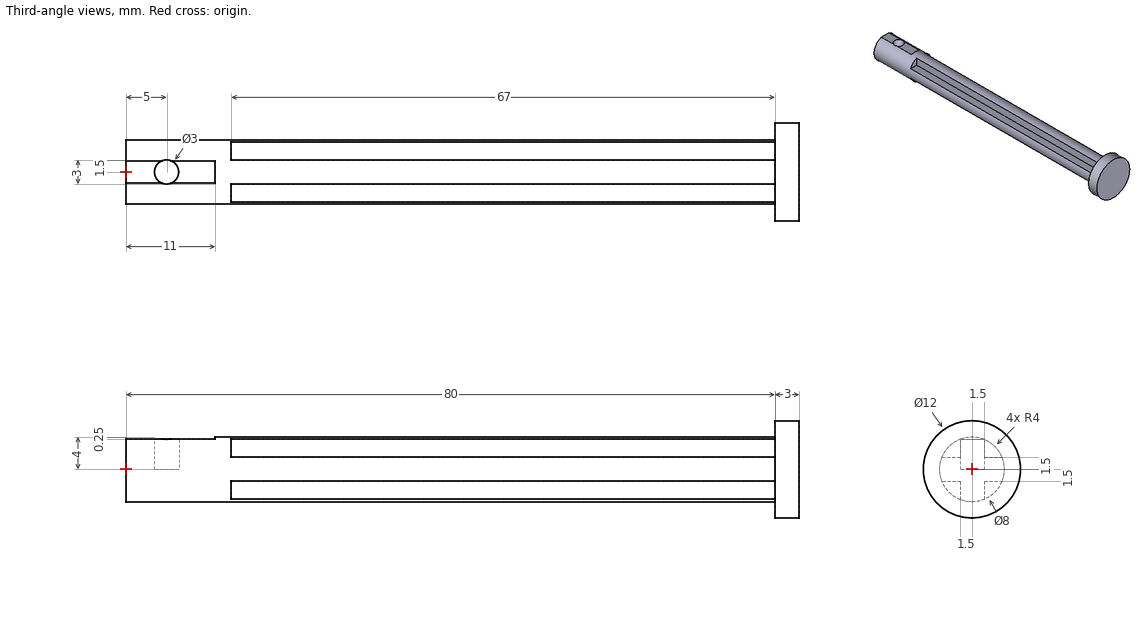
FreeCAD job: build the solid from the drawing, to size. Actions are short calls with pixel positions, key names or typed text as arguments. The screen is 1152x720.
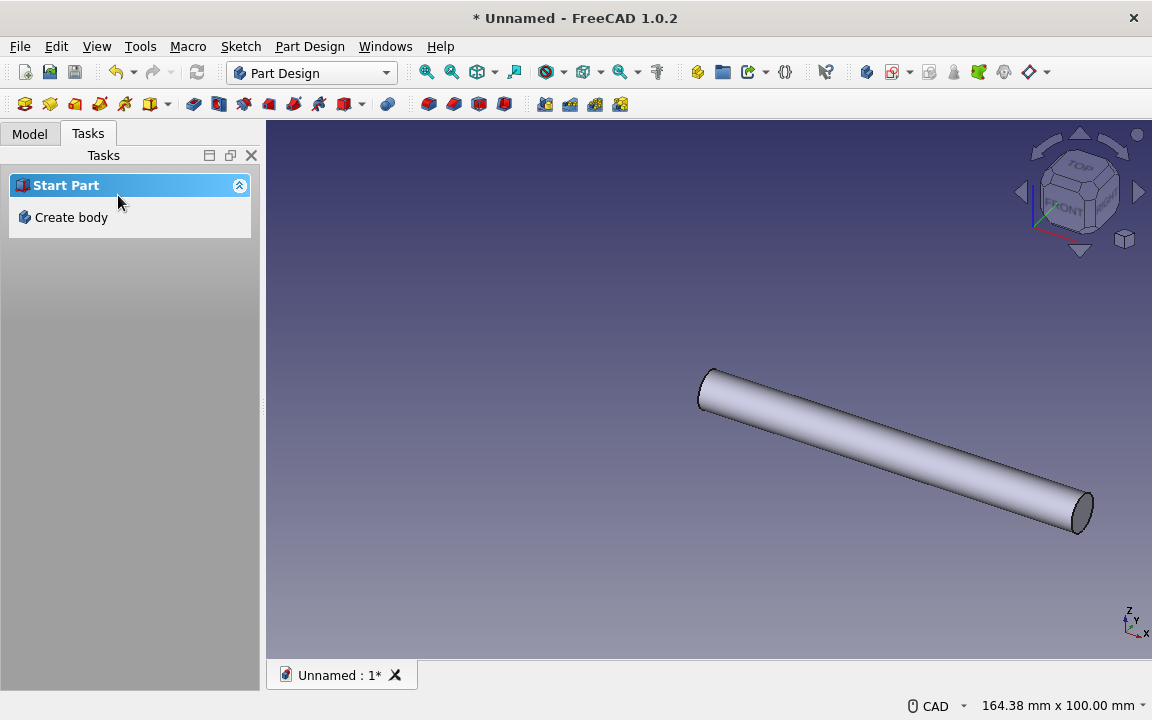
click(427, 72)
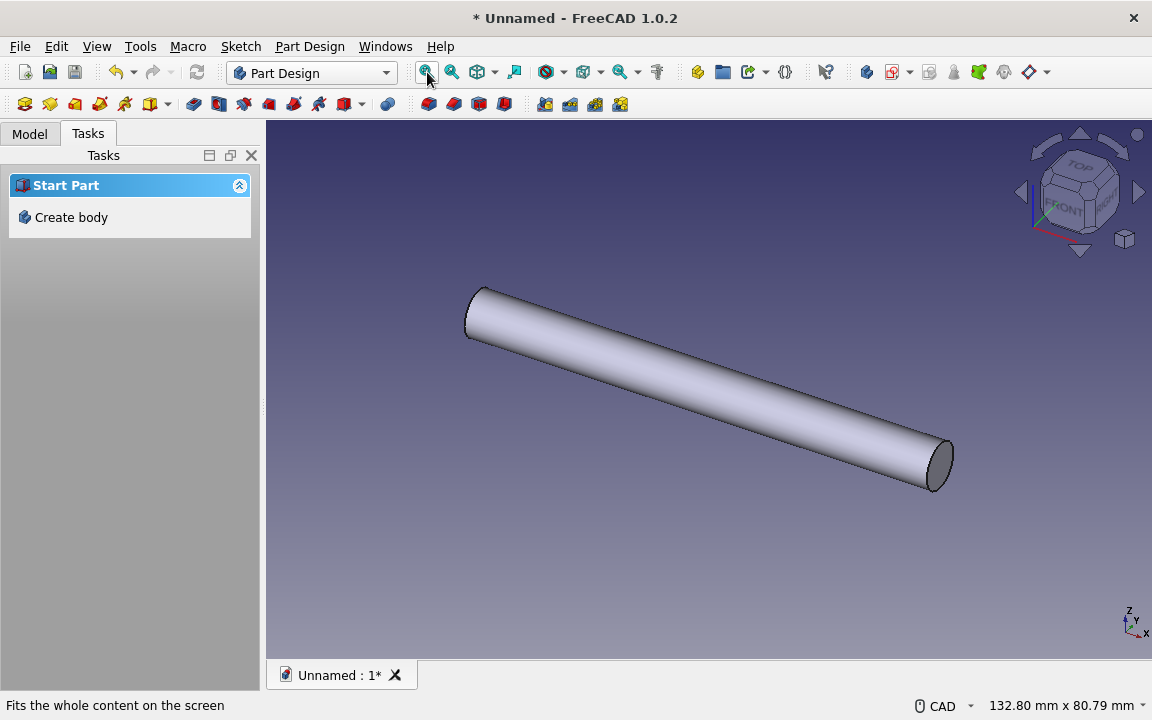
click(30, 134)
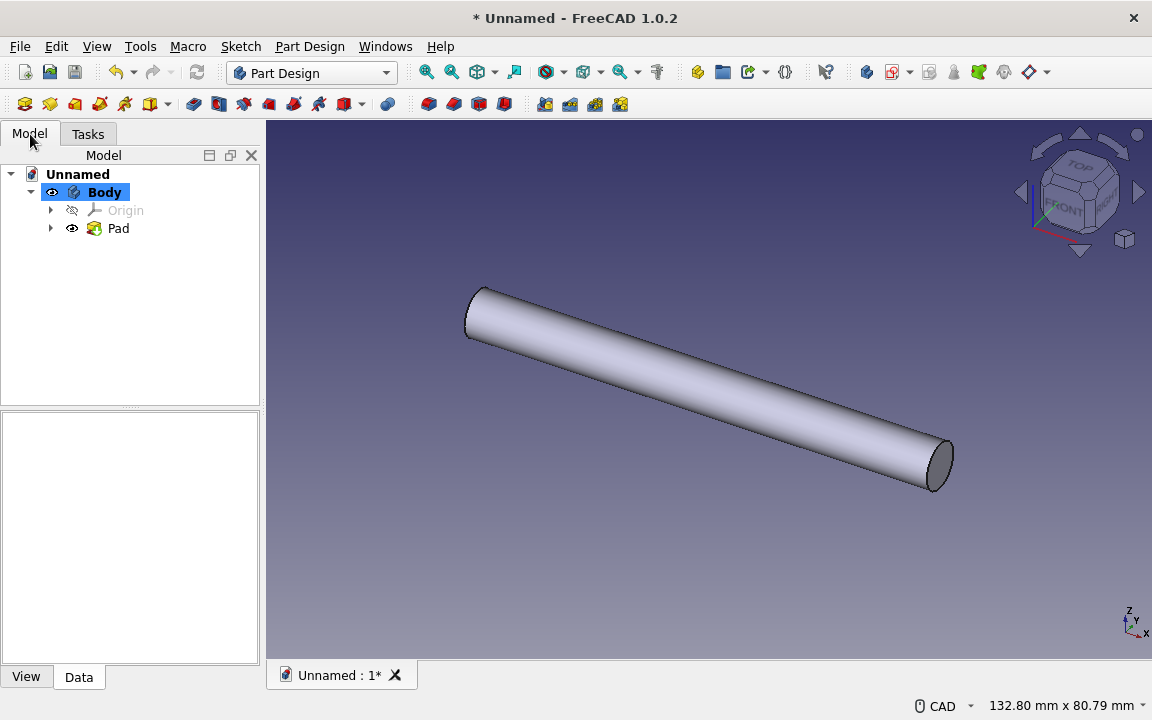
click(51, 210)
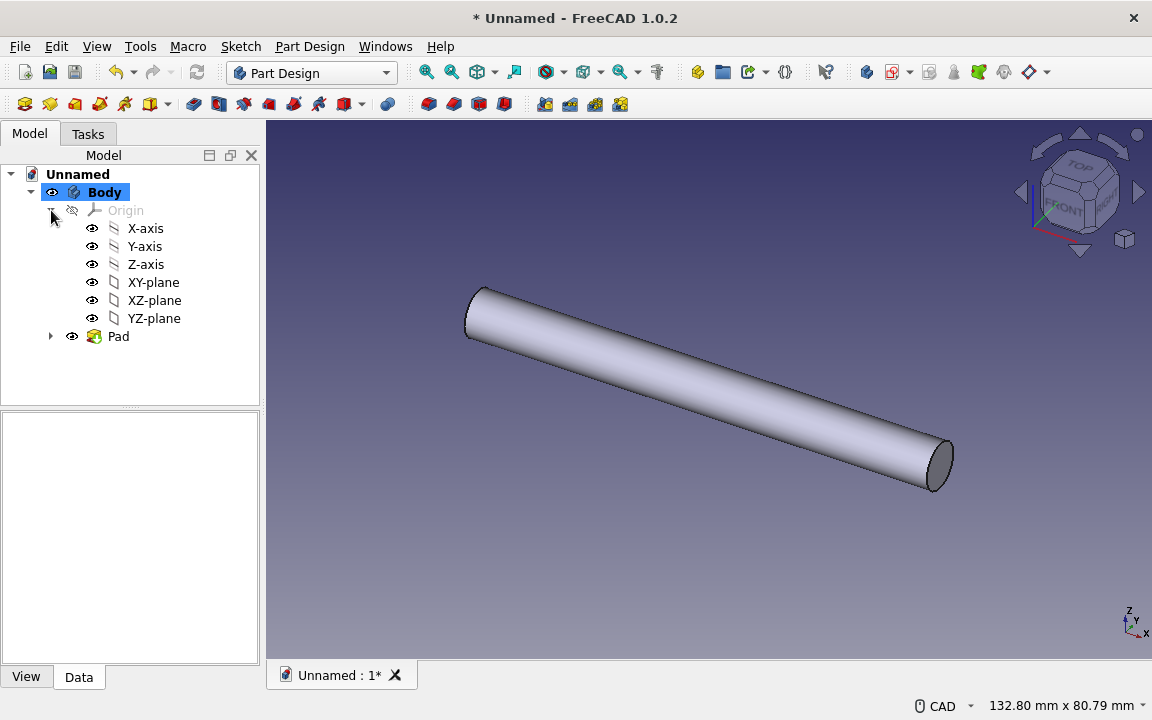
click(137, 318)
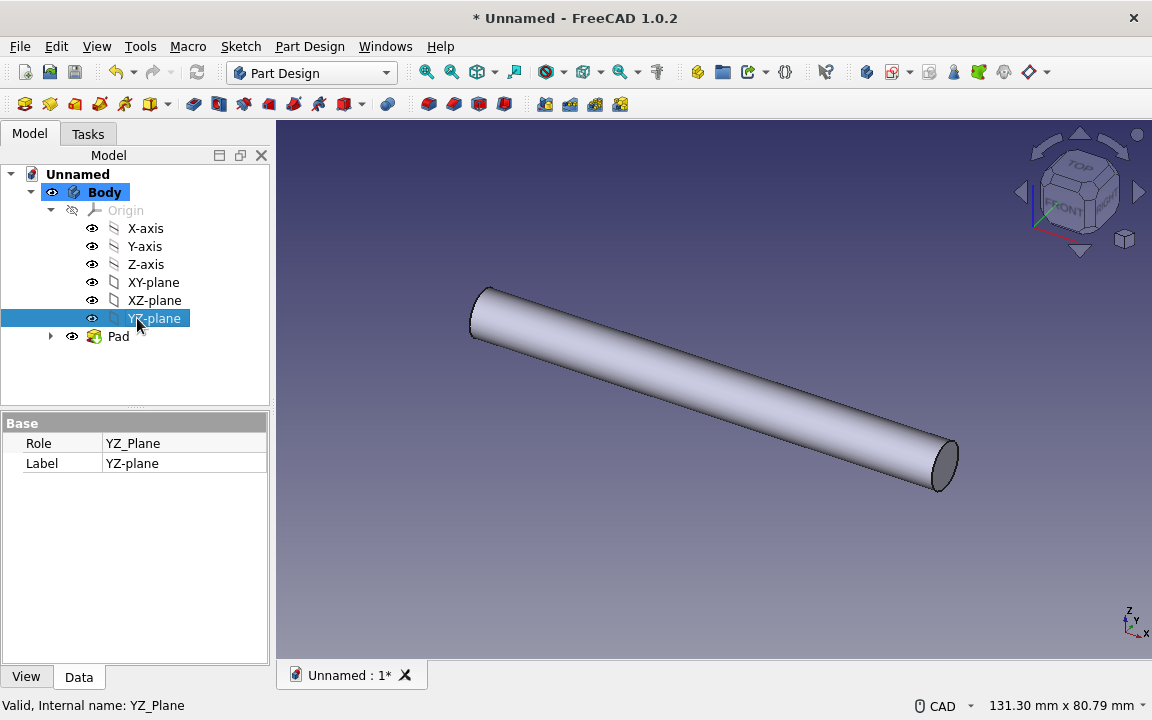
click(1028, 72)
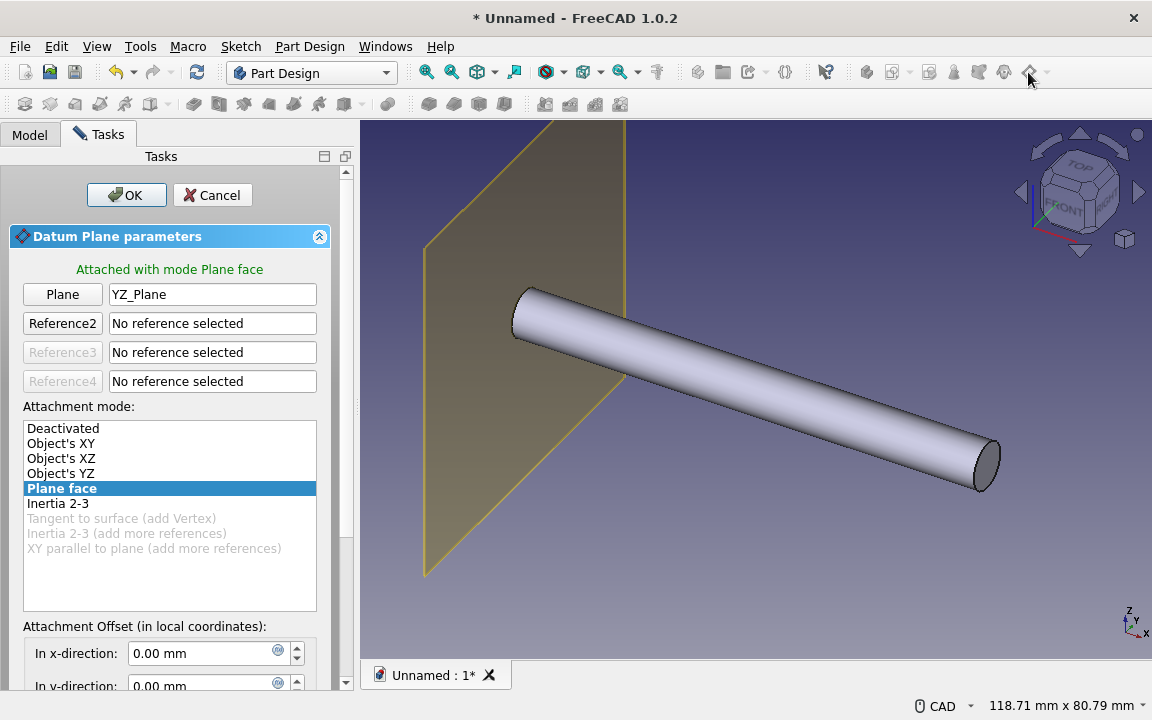
scroll(346, 428, down, 2)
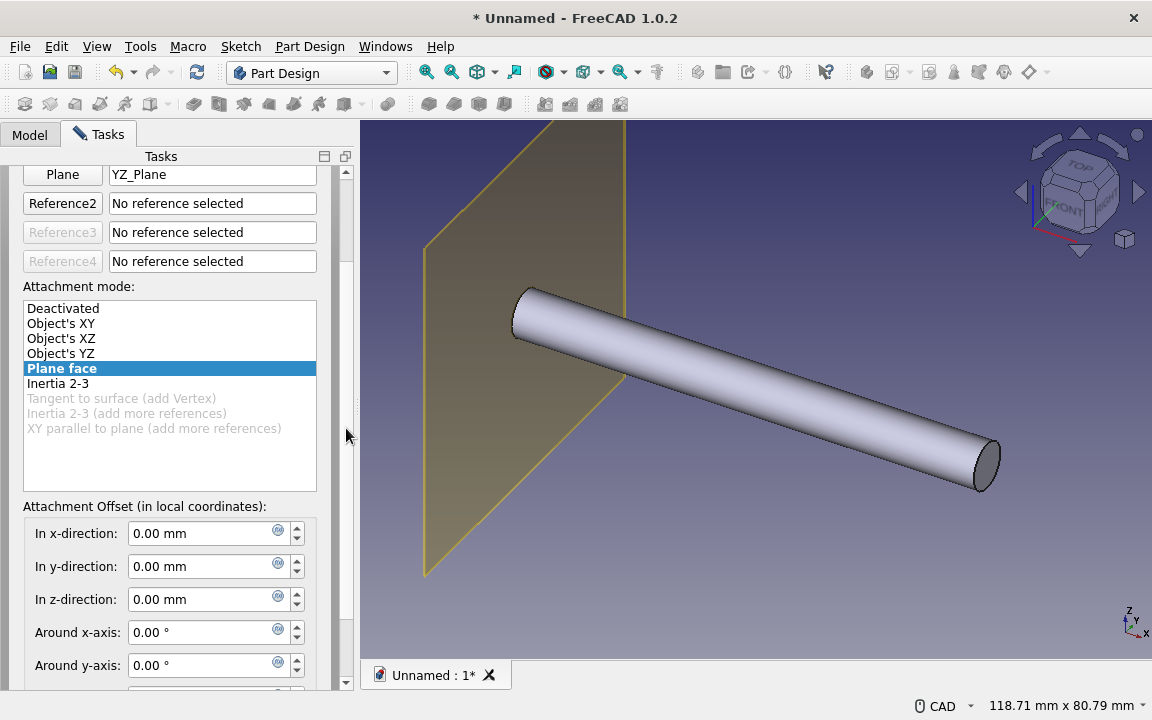
triple_click(210, 600)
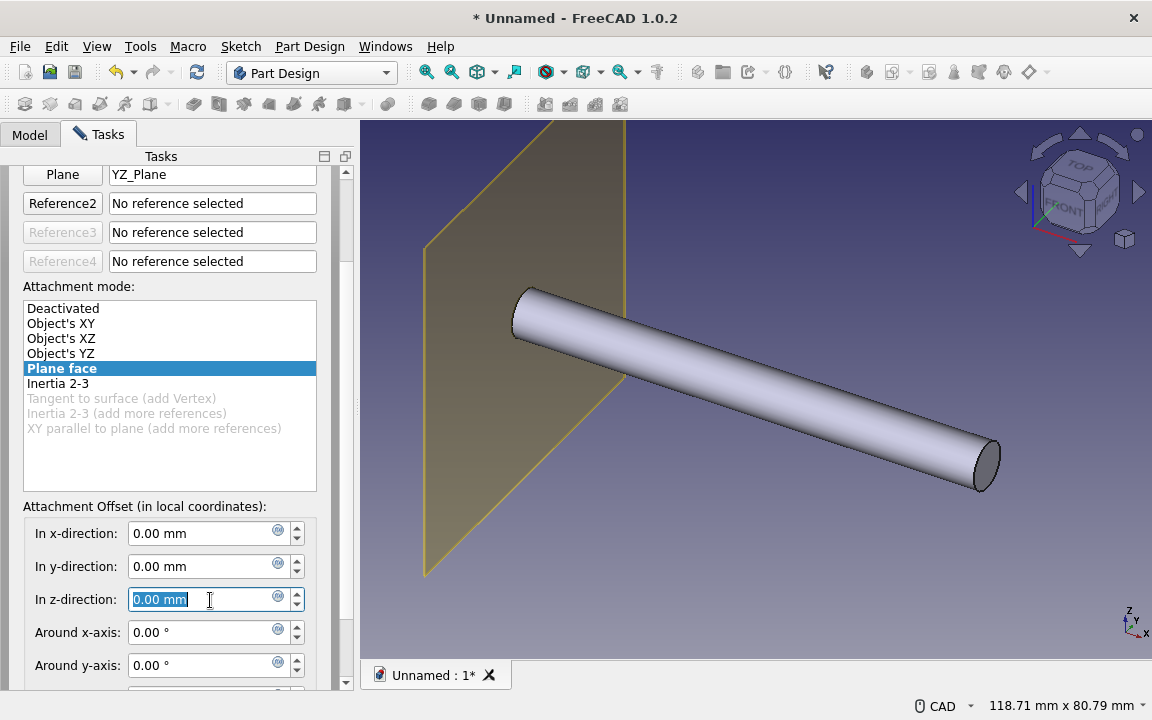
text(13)
key(Tab)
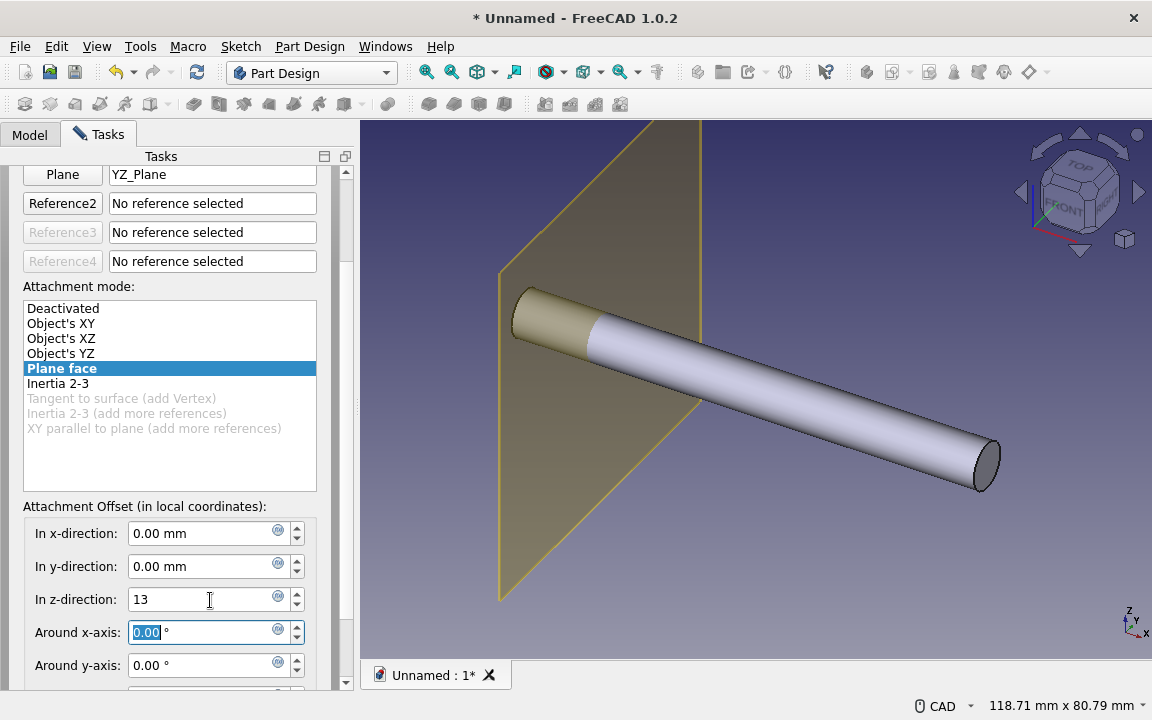
scroll(346, 428, up, 3)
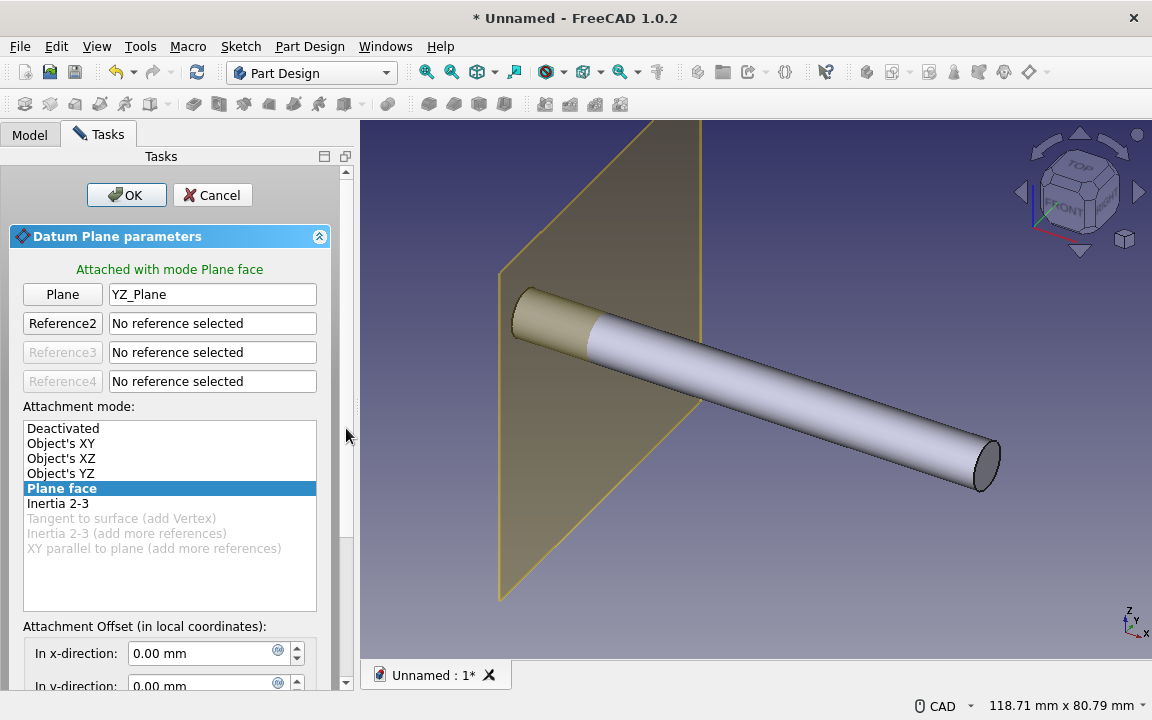
click(127, 195)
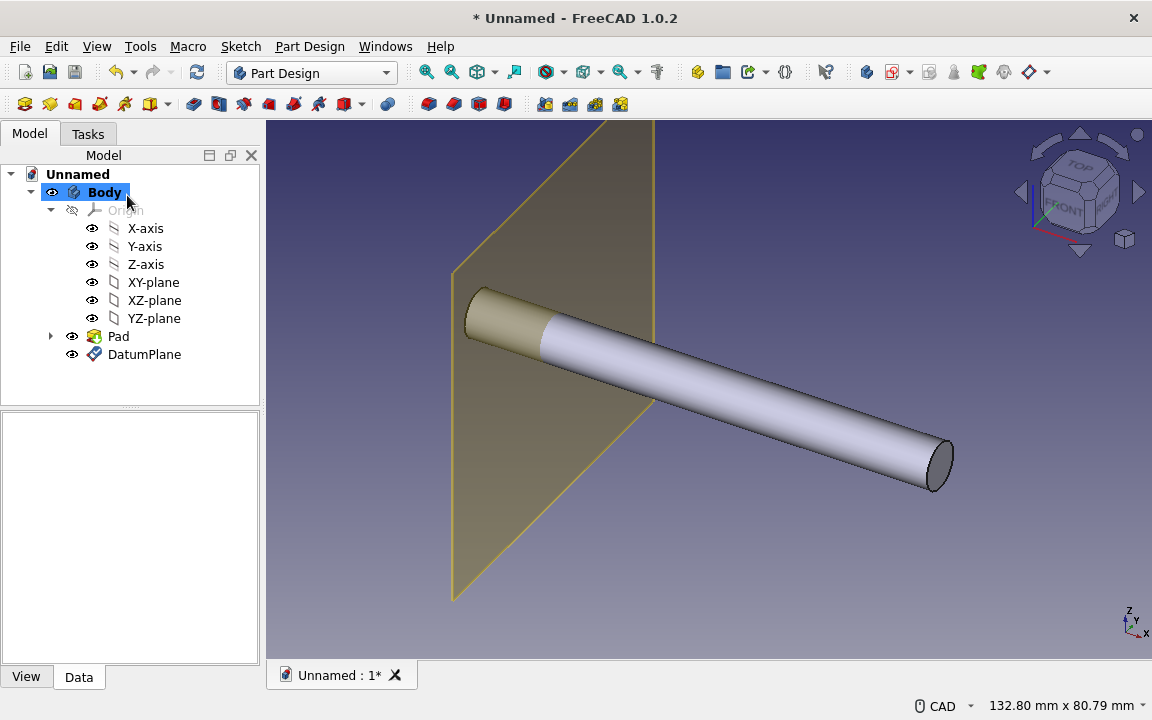
click(117, 354)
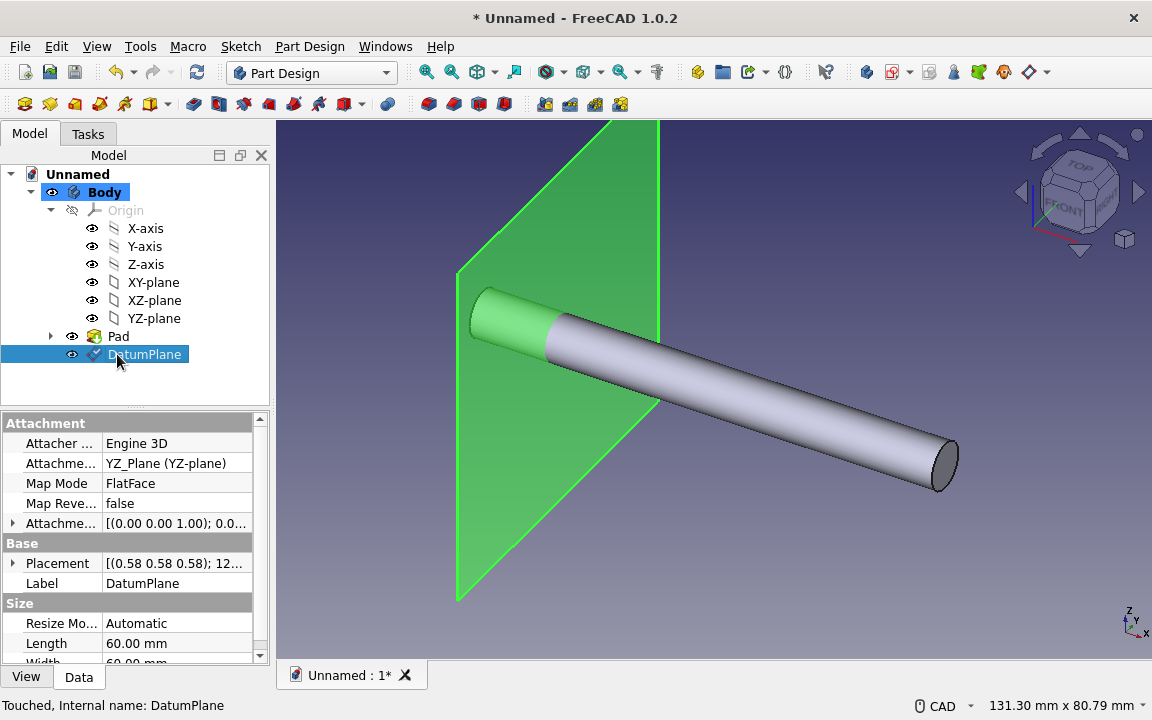
click(892, 72)